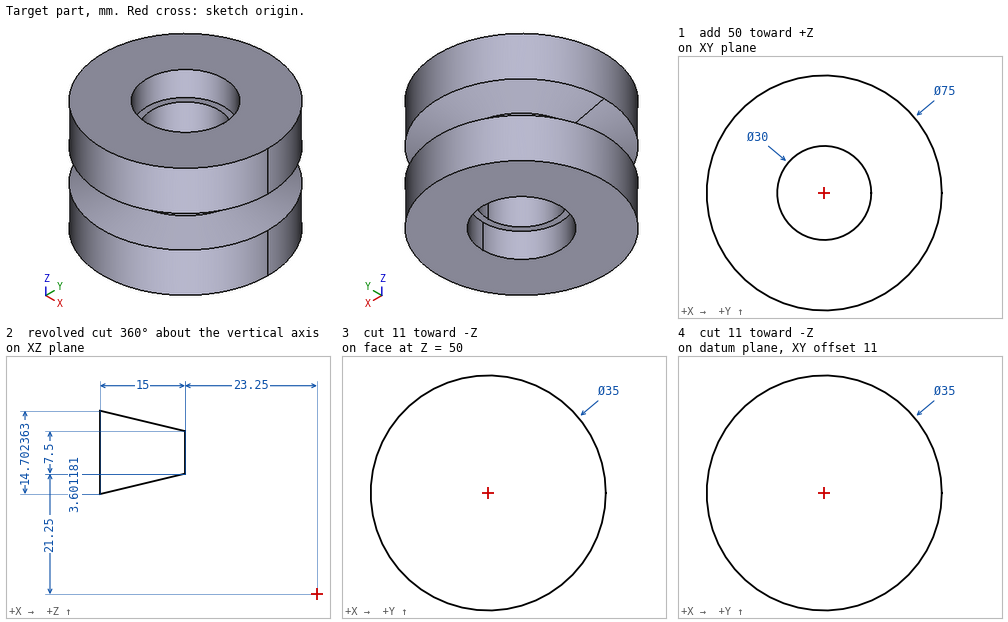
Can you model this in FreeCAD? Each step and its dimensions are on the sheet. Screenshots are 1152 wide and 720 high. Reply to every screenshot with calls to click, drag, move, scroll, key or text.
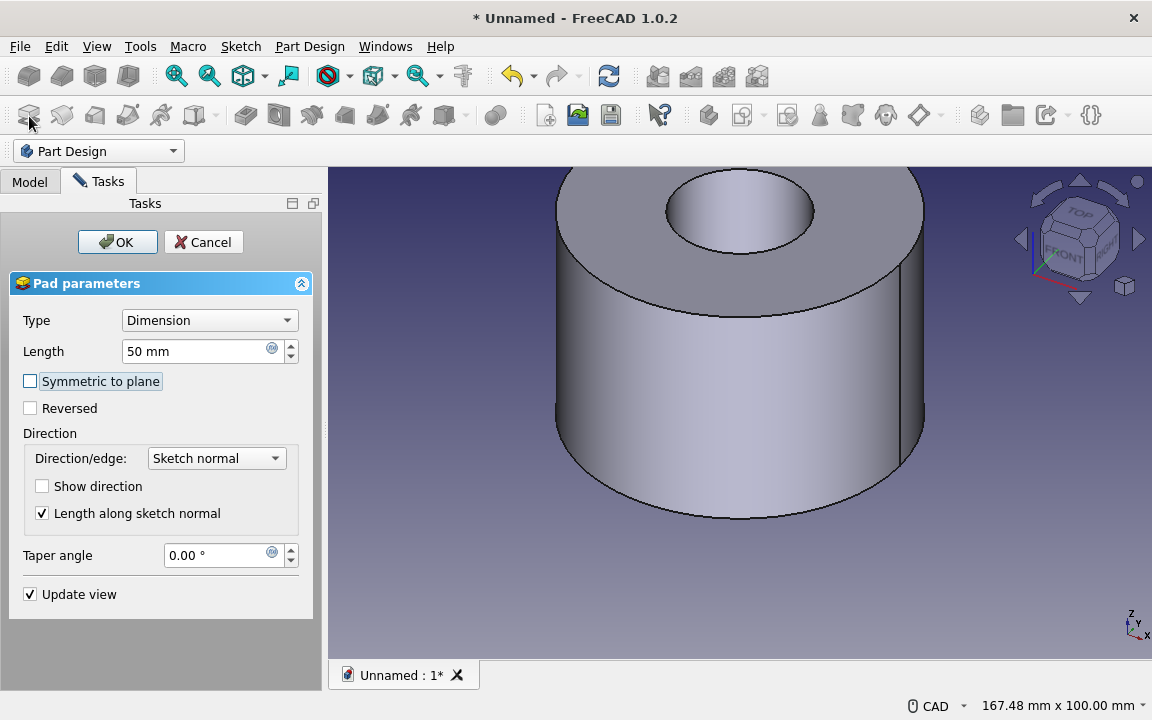
click(118, 242)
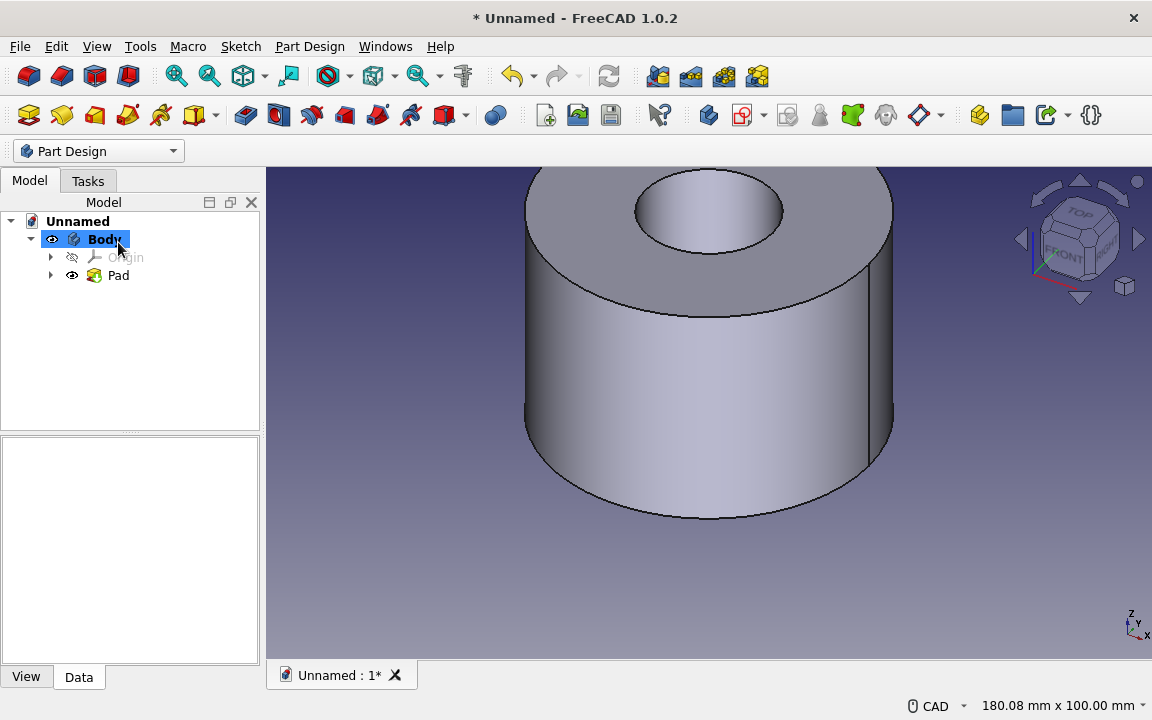
key(v)
key(f)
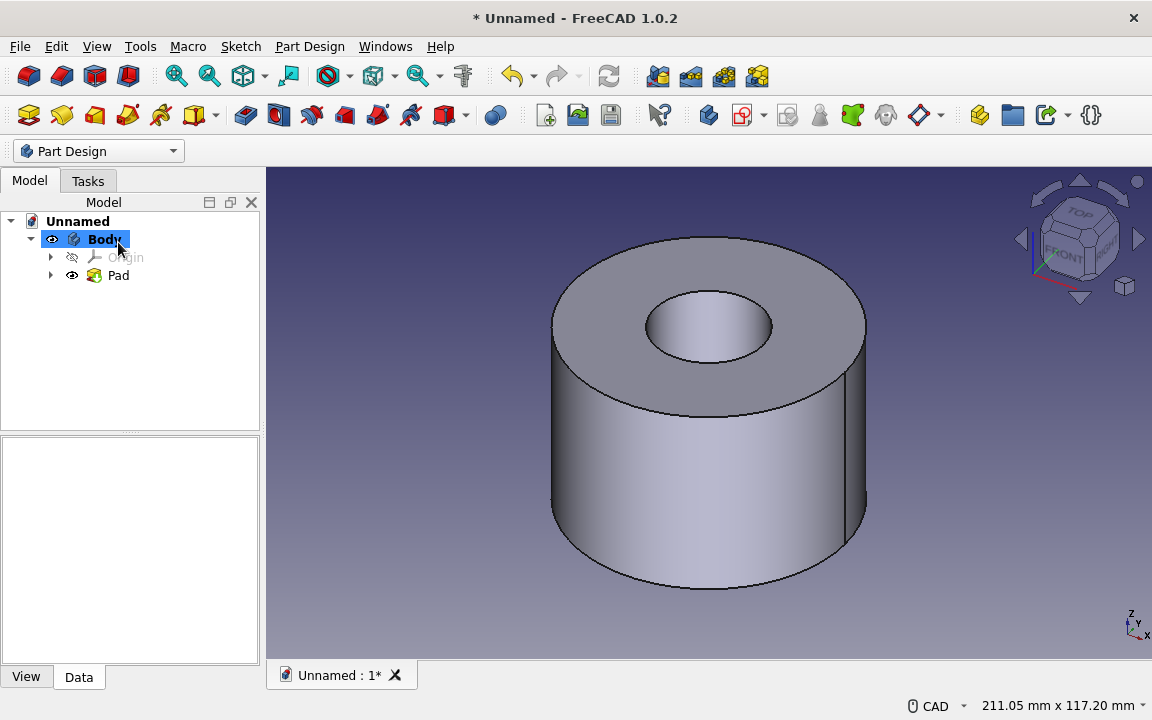
click(742, 116)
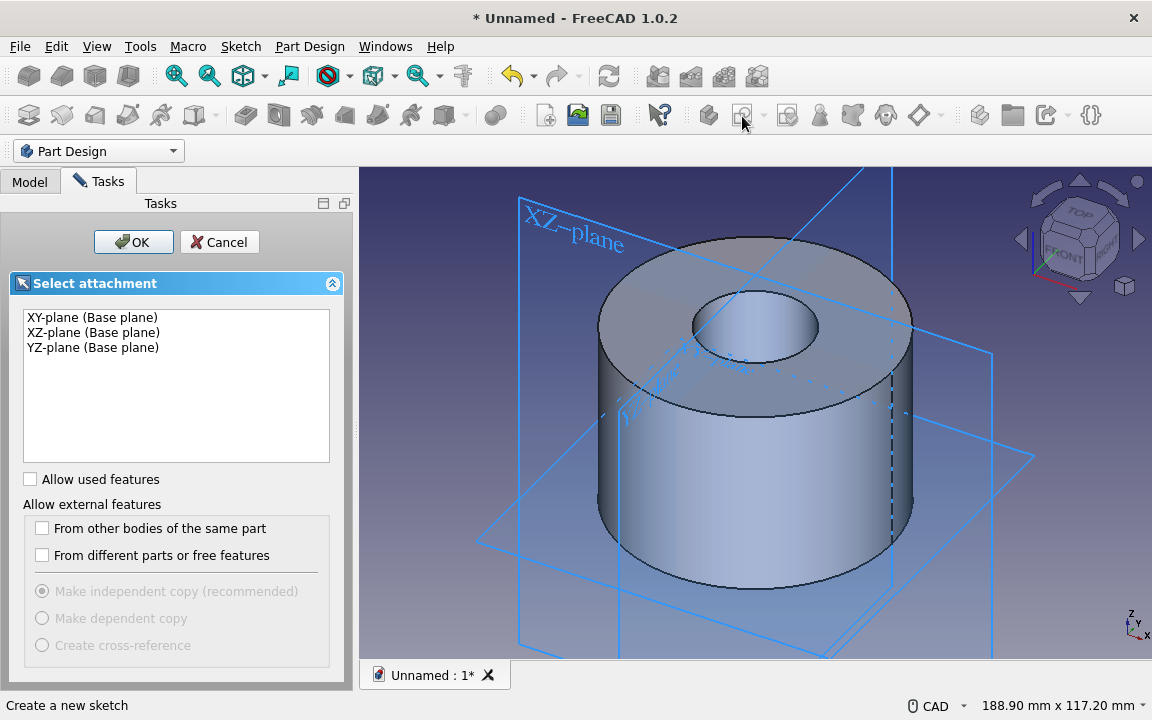
click(84, 332)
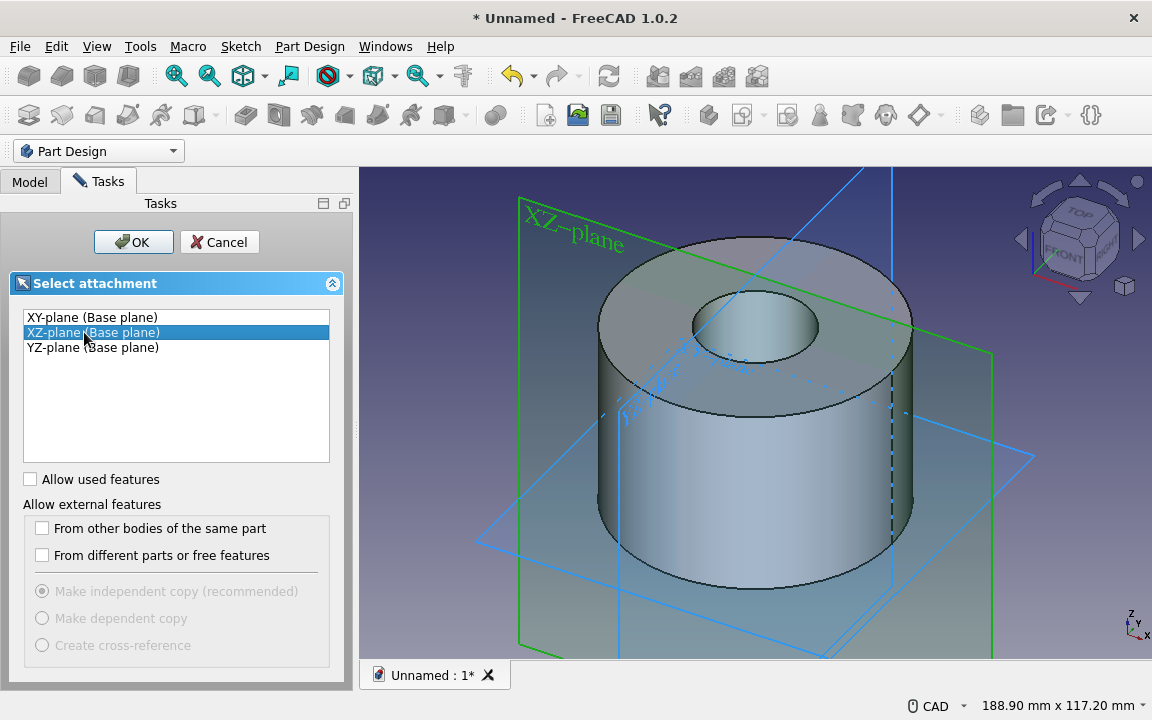
click(134, 242)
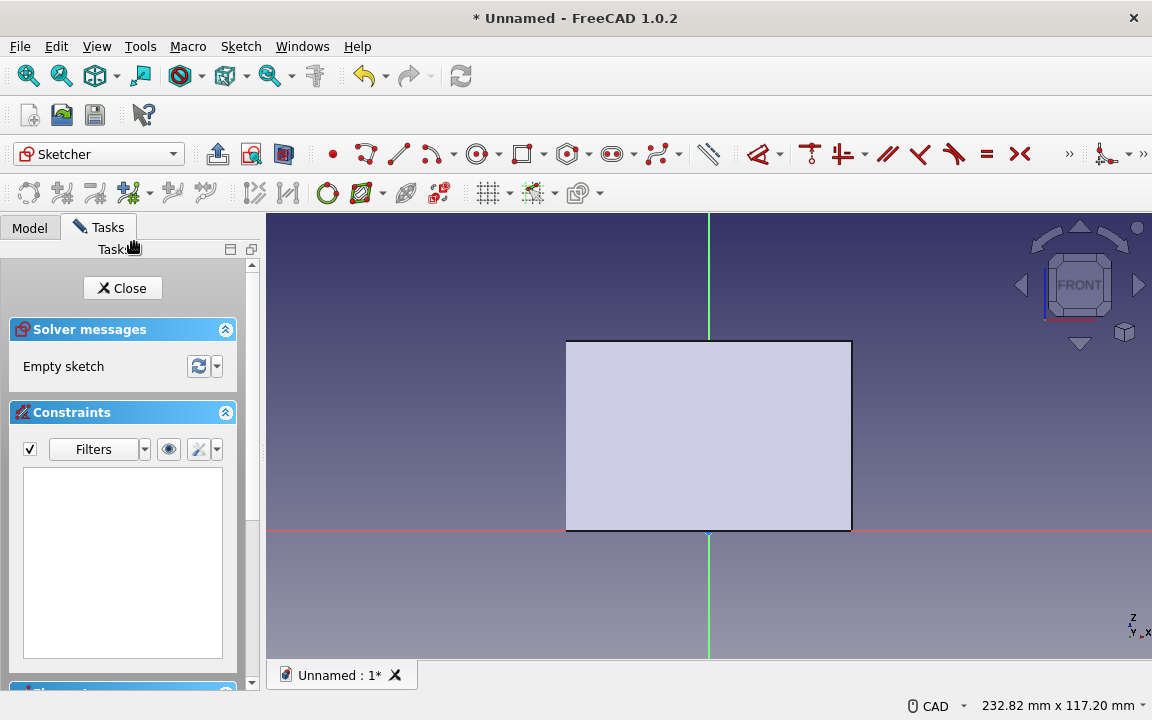
key(q)
key(s)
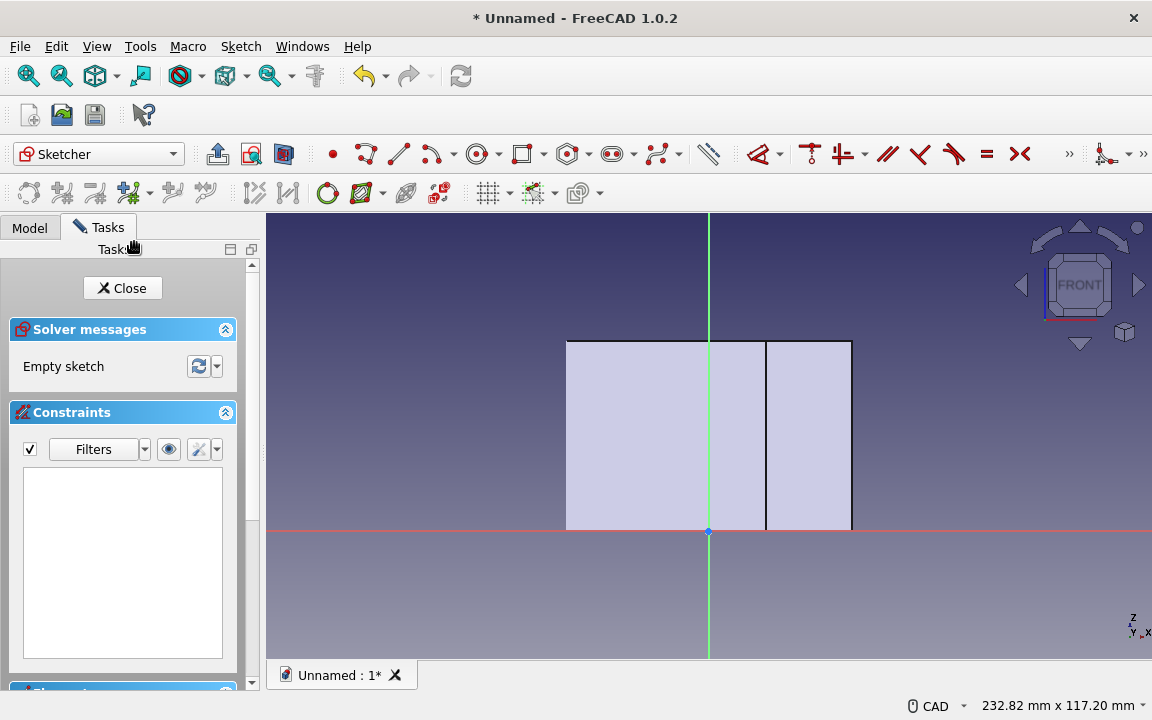
scroll(580, 436, up, 8)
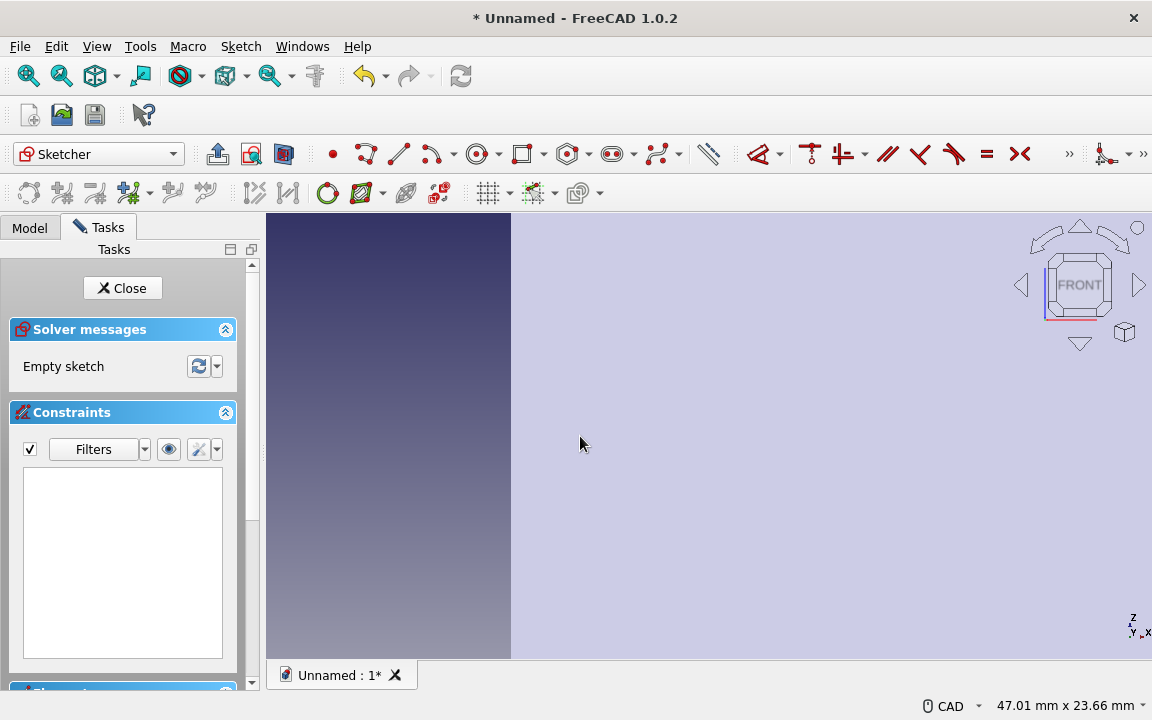
click(366, 154)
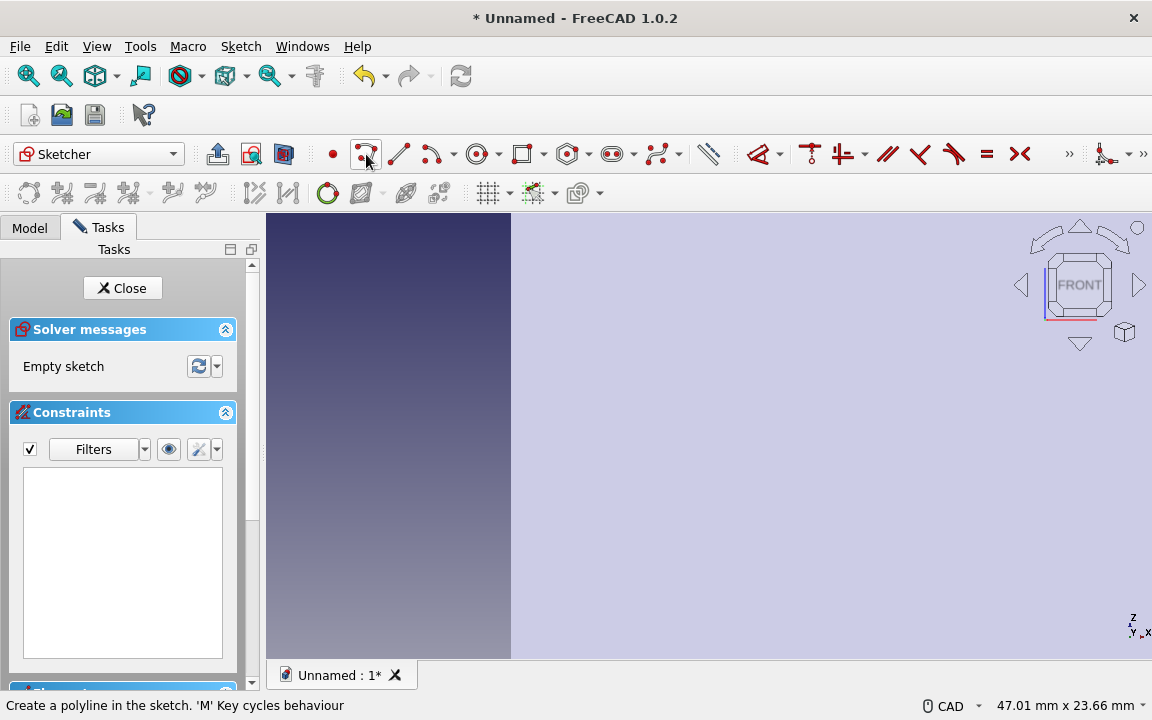
click(779, 505)
click(496, 573)
click(496, 295)
click(779, 363)
click(779, 506)
key(Escape)
key(Escape)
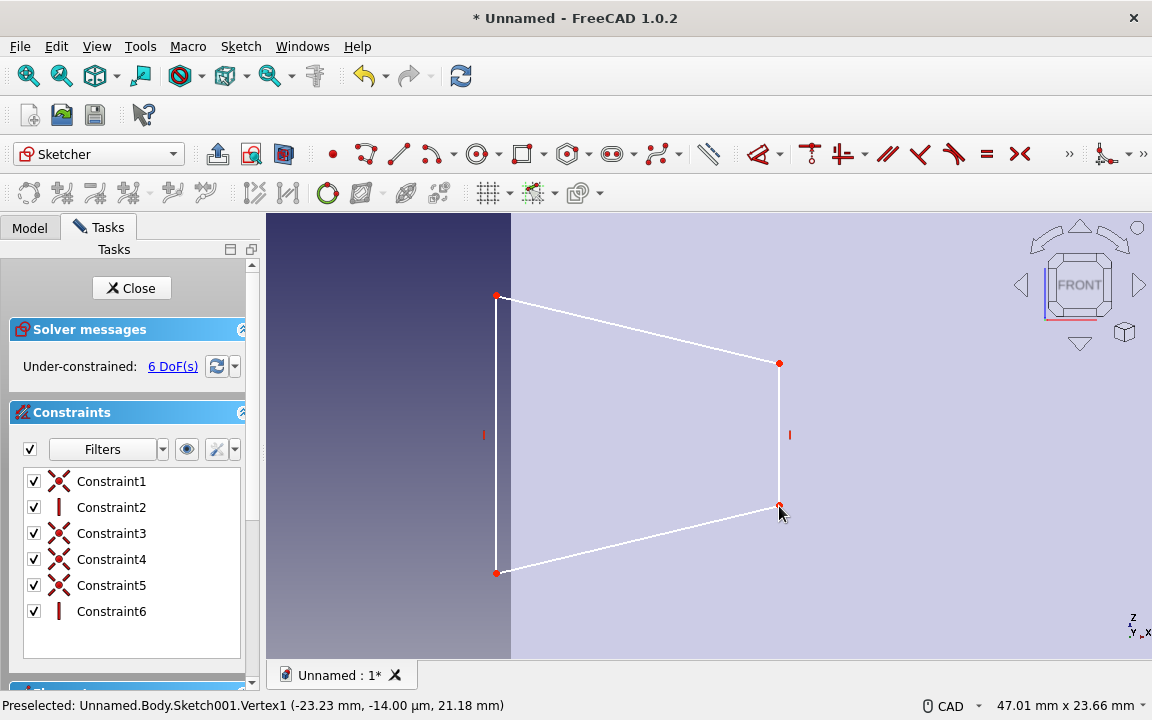
key(d)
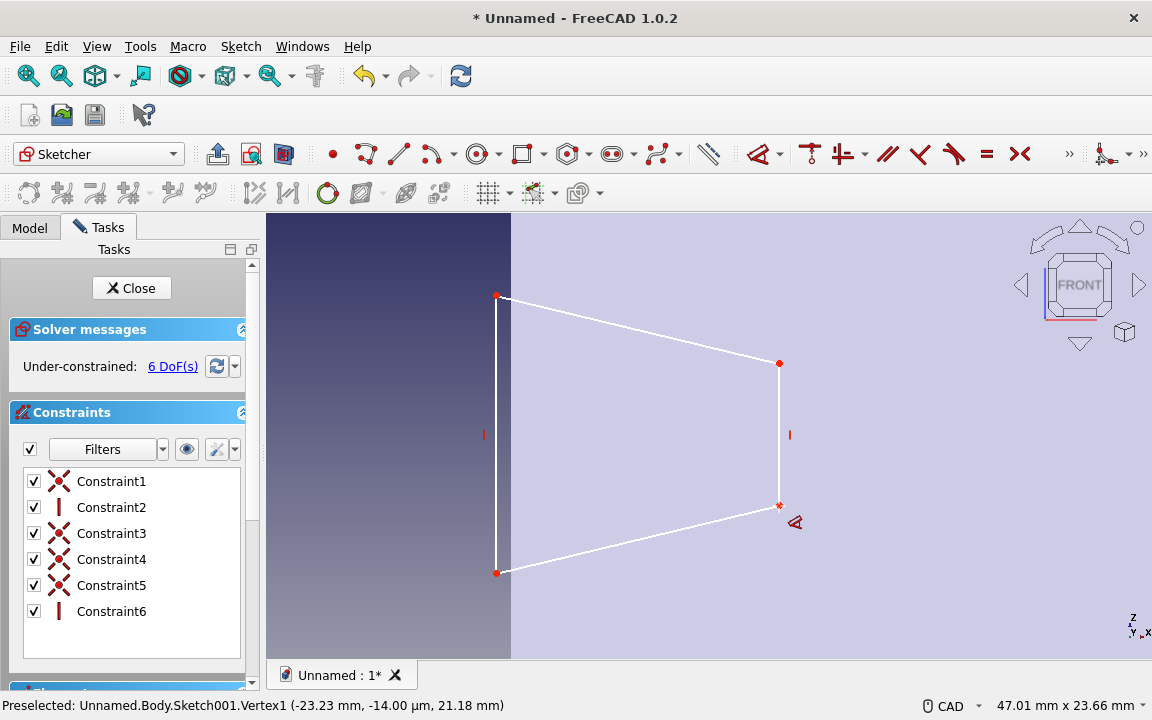
click(779, 407)
click(813, 435)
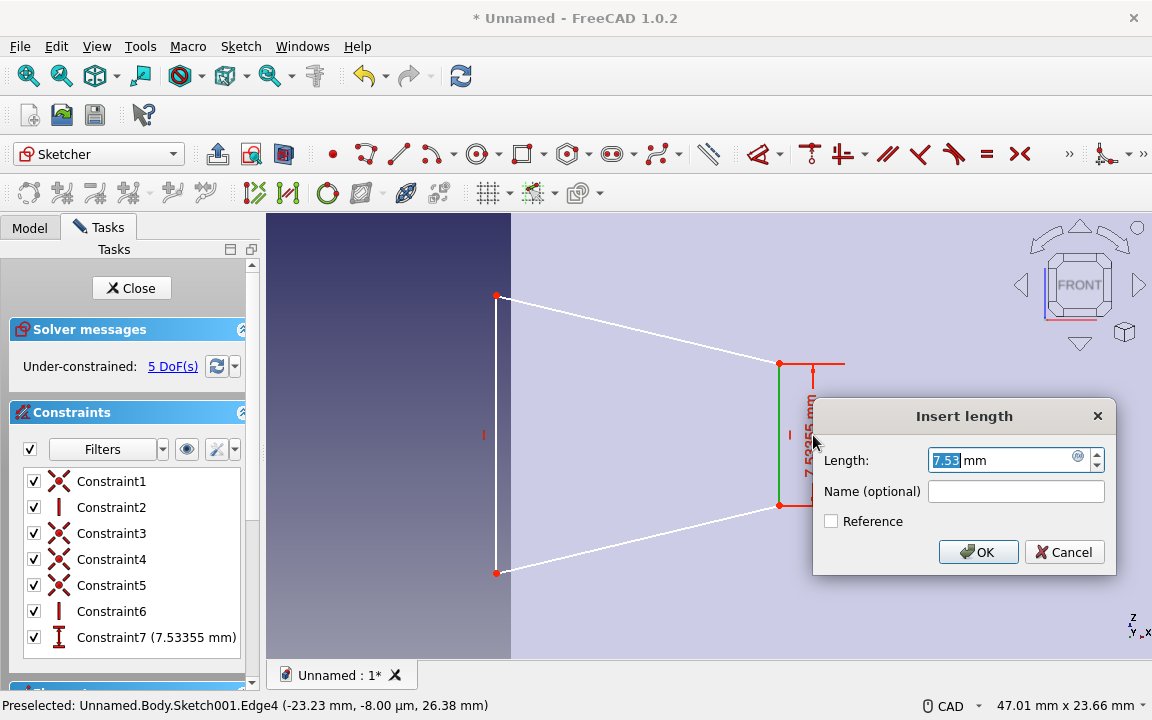
text(7.5)
key(Return)